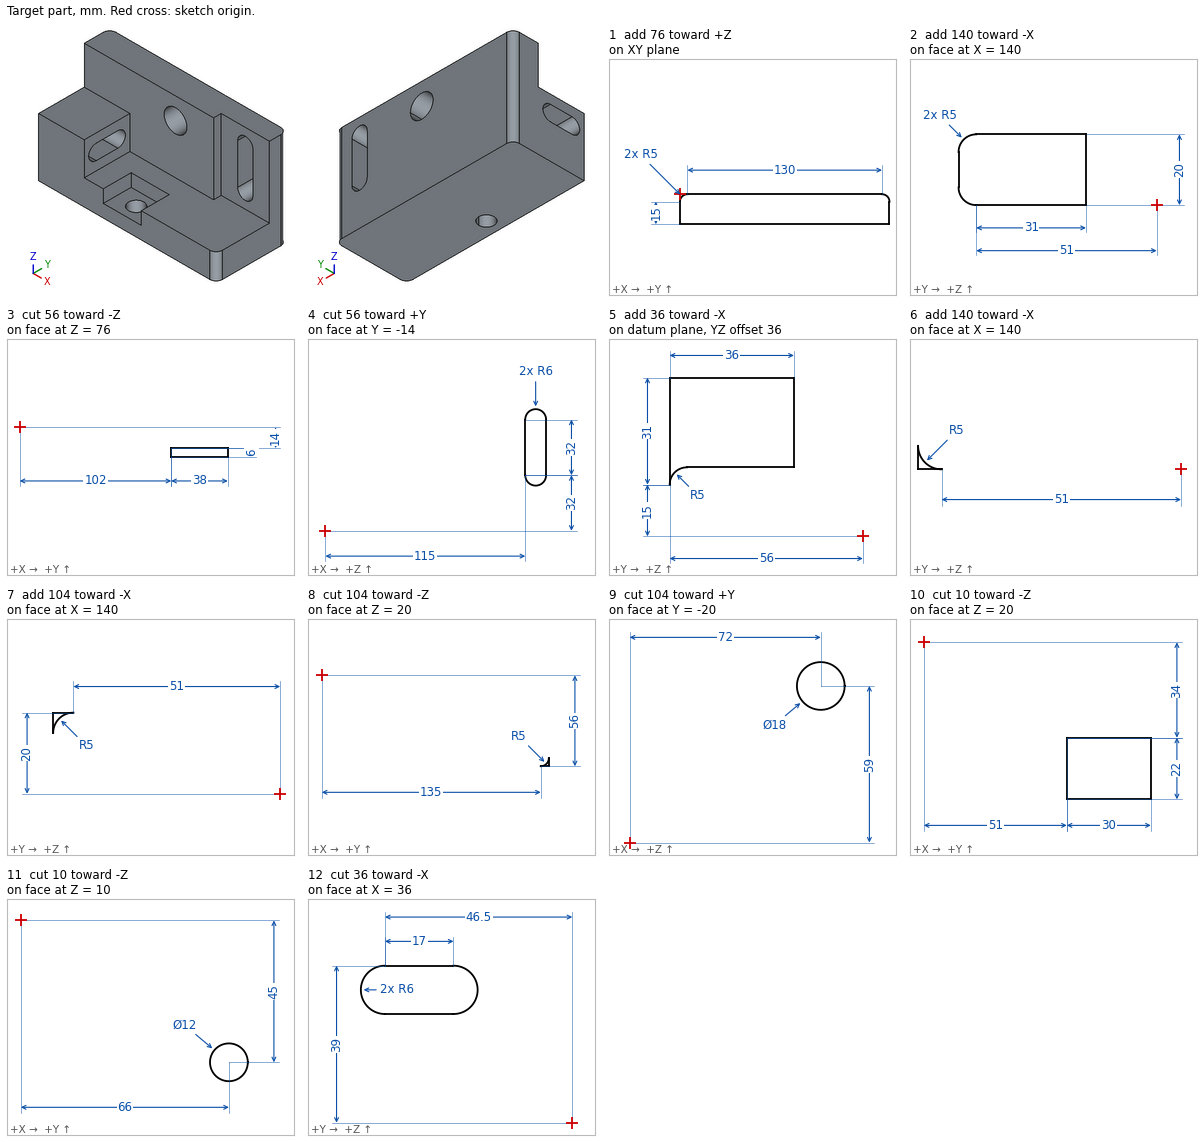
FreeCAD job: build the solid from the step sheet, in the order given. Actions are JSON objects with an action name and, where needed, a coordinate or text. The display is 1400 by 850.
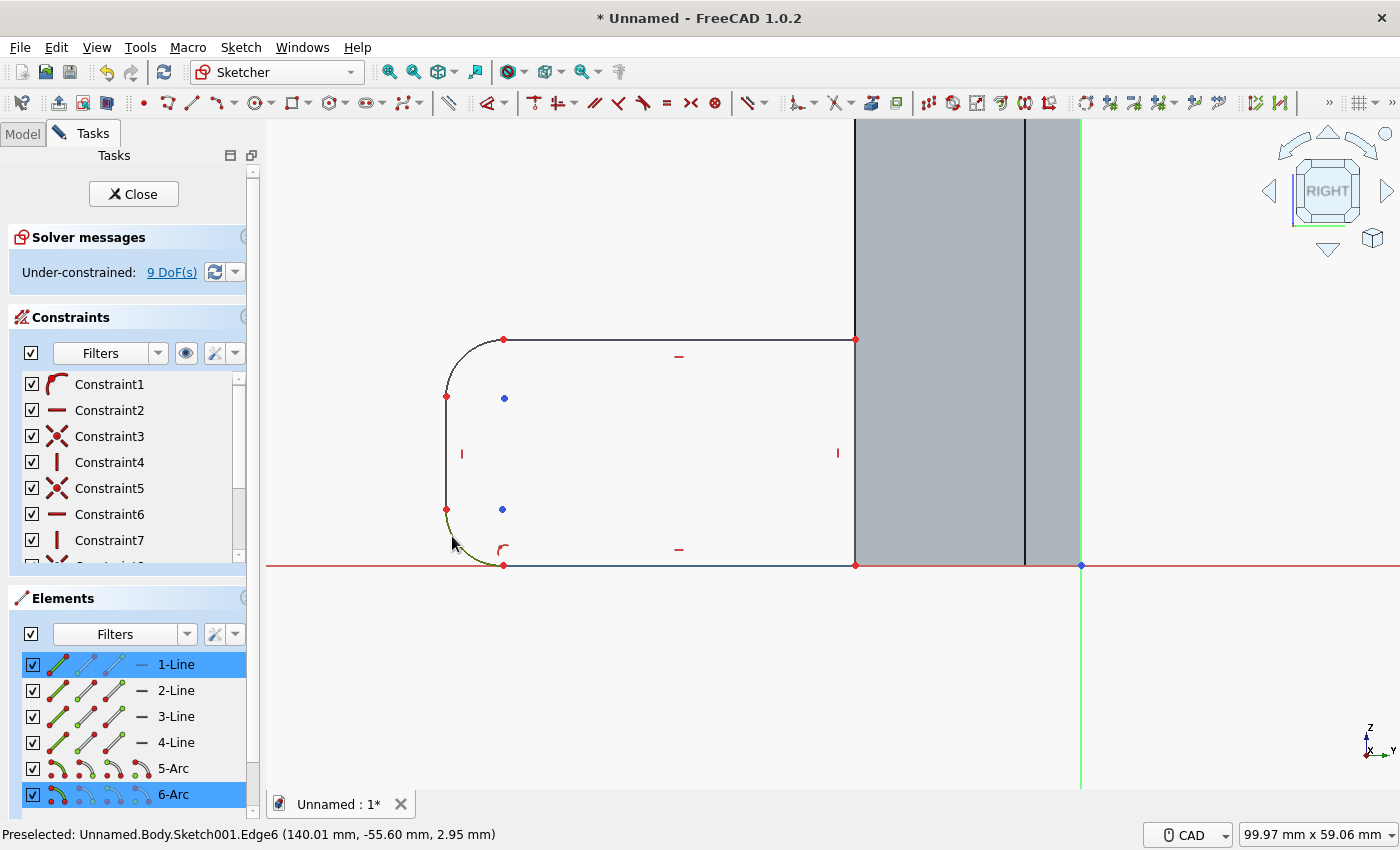
{"action": "key", "text": "t"}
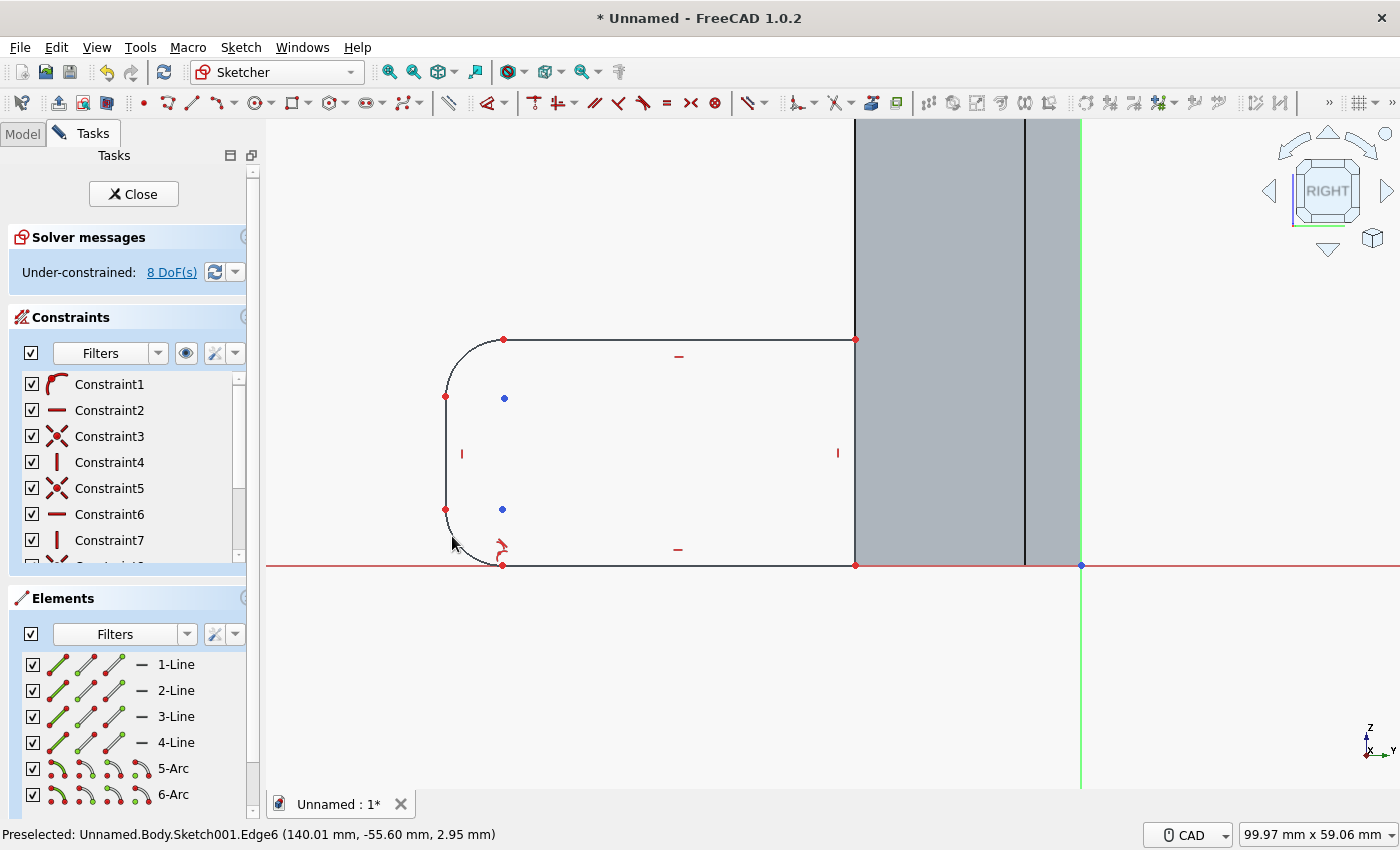
{"action": "left_click", "coordinate": [749, 340]}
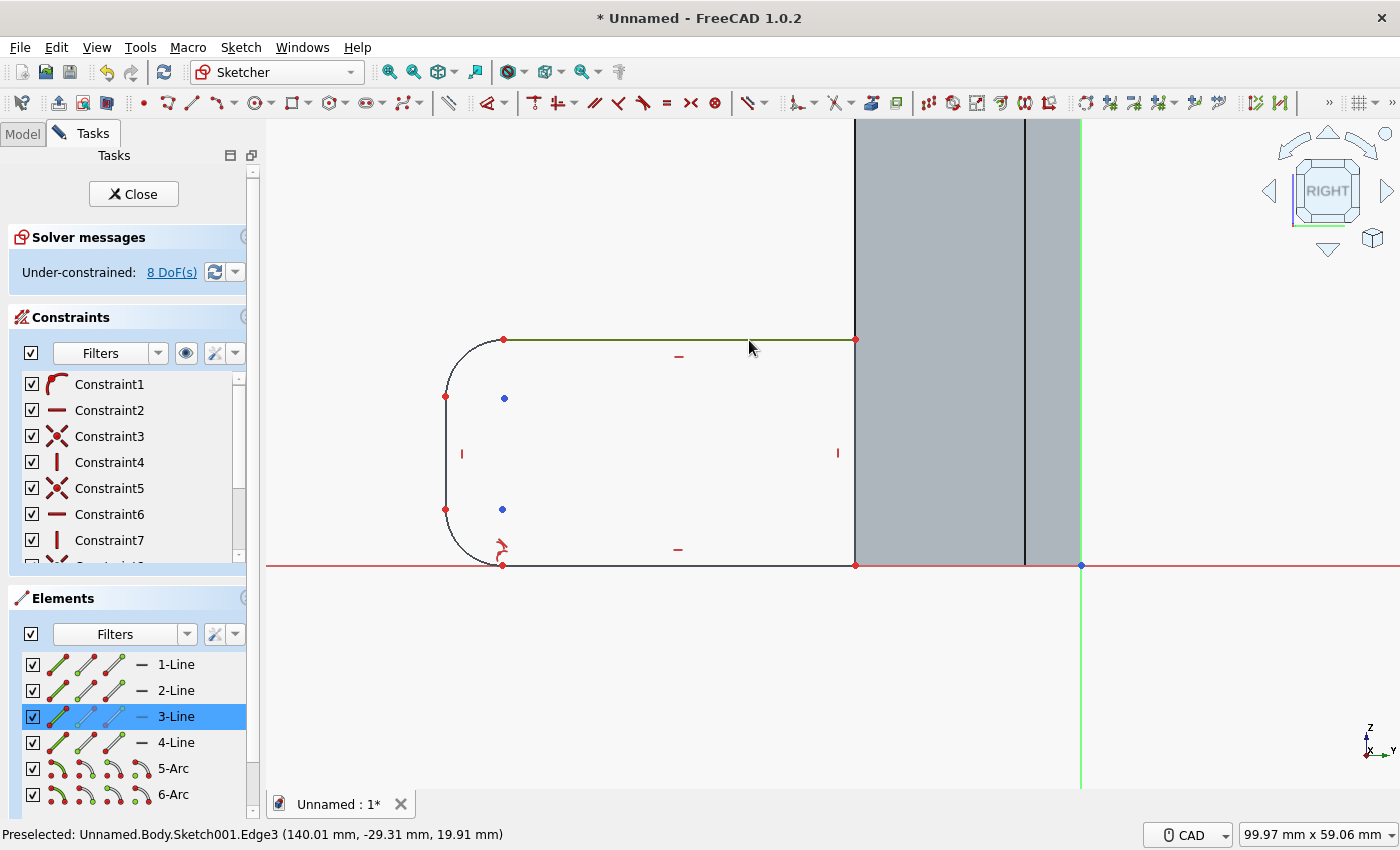
{"action": "left_click", "coordinate": [477, 347]}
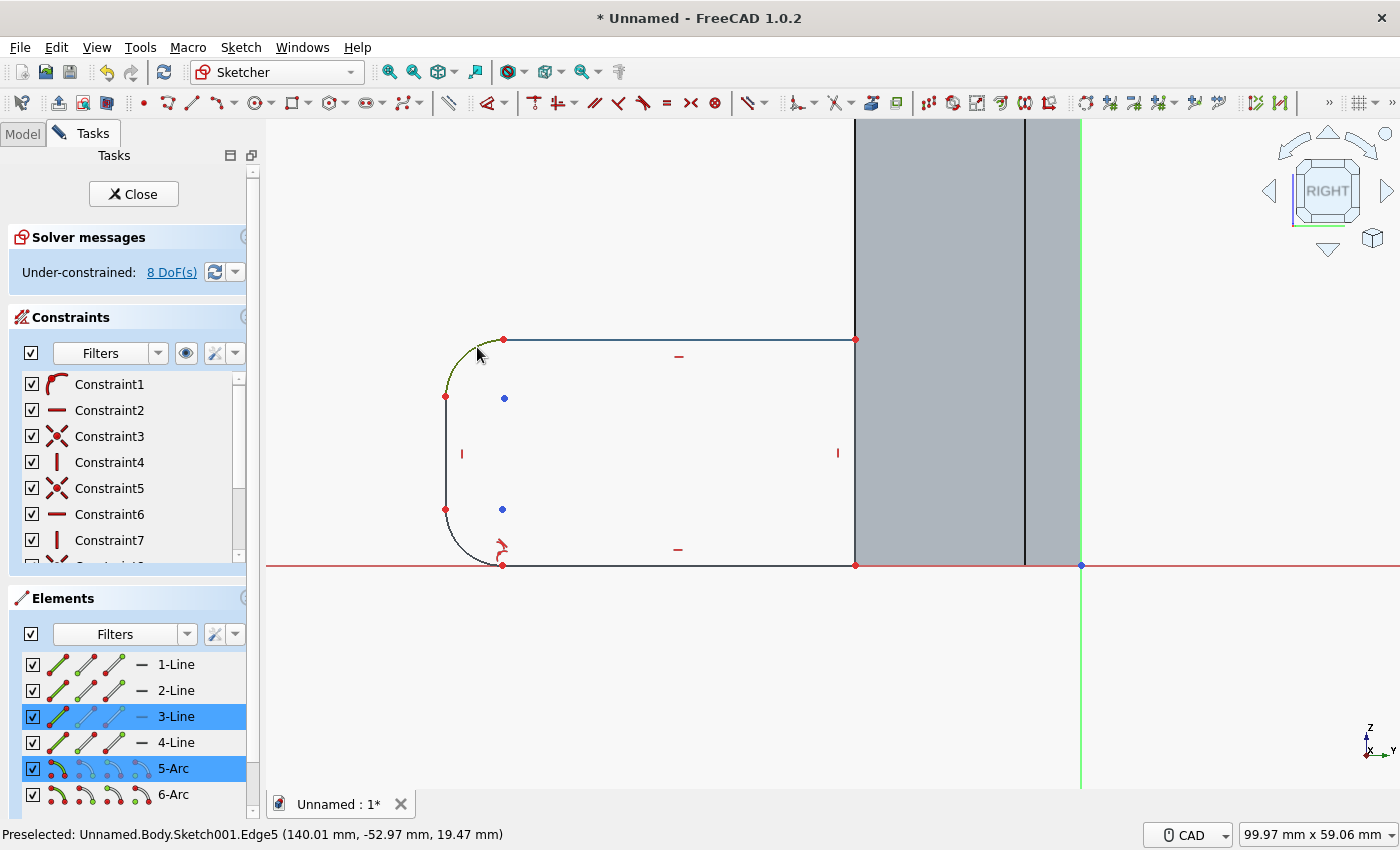
{"action": "left_click", "coordinate": [644, 104]}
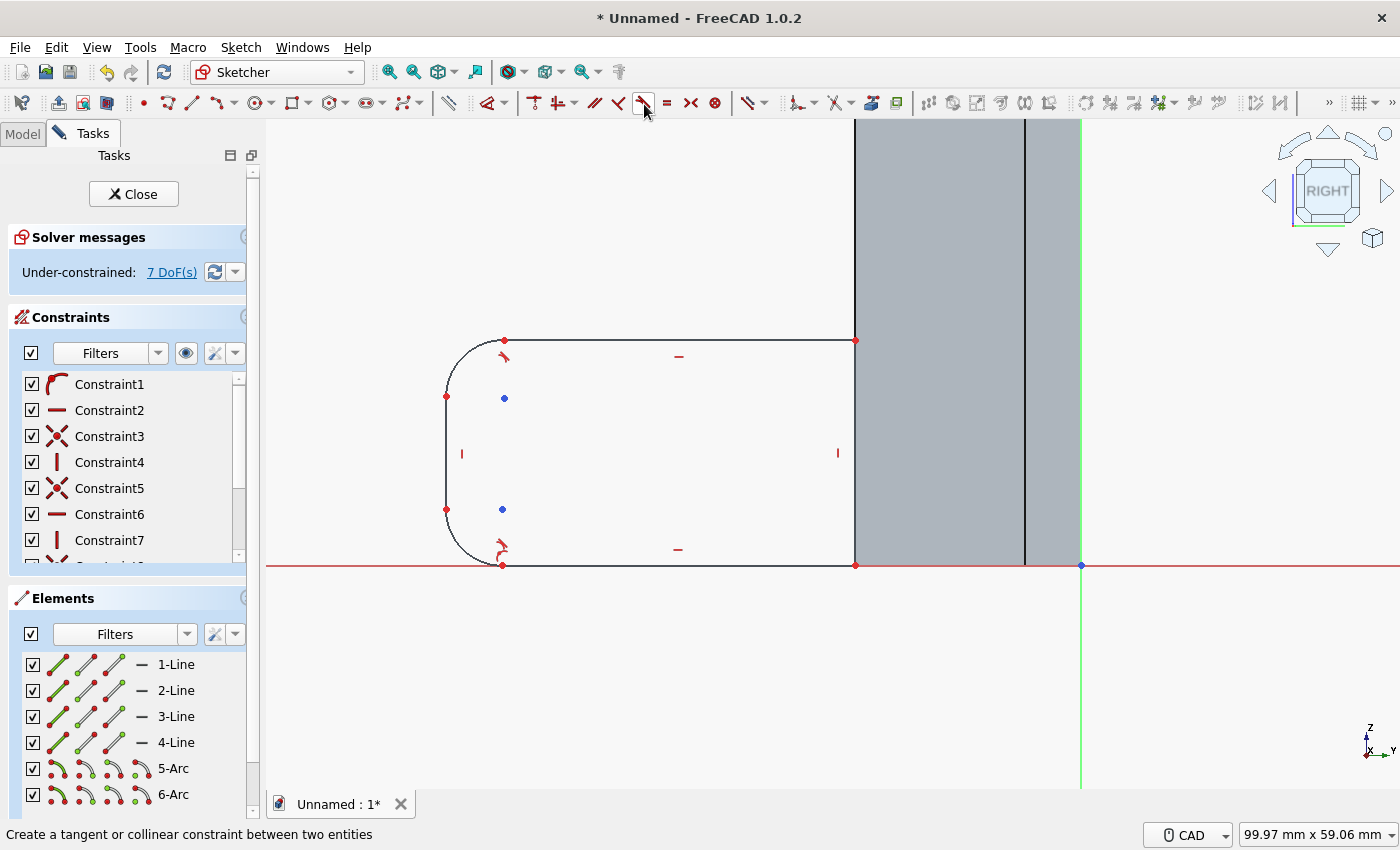
{"action": "left_click", "coordinate": [446, 431]}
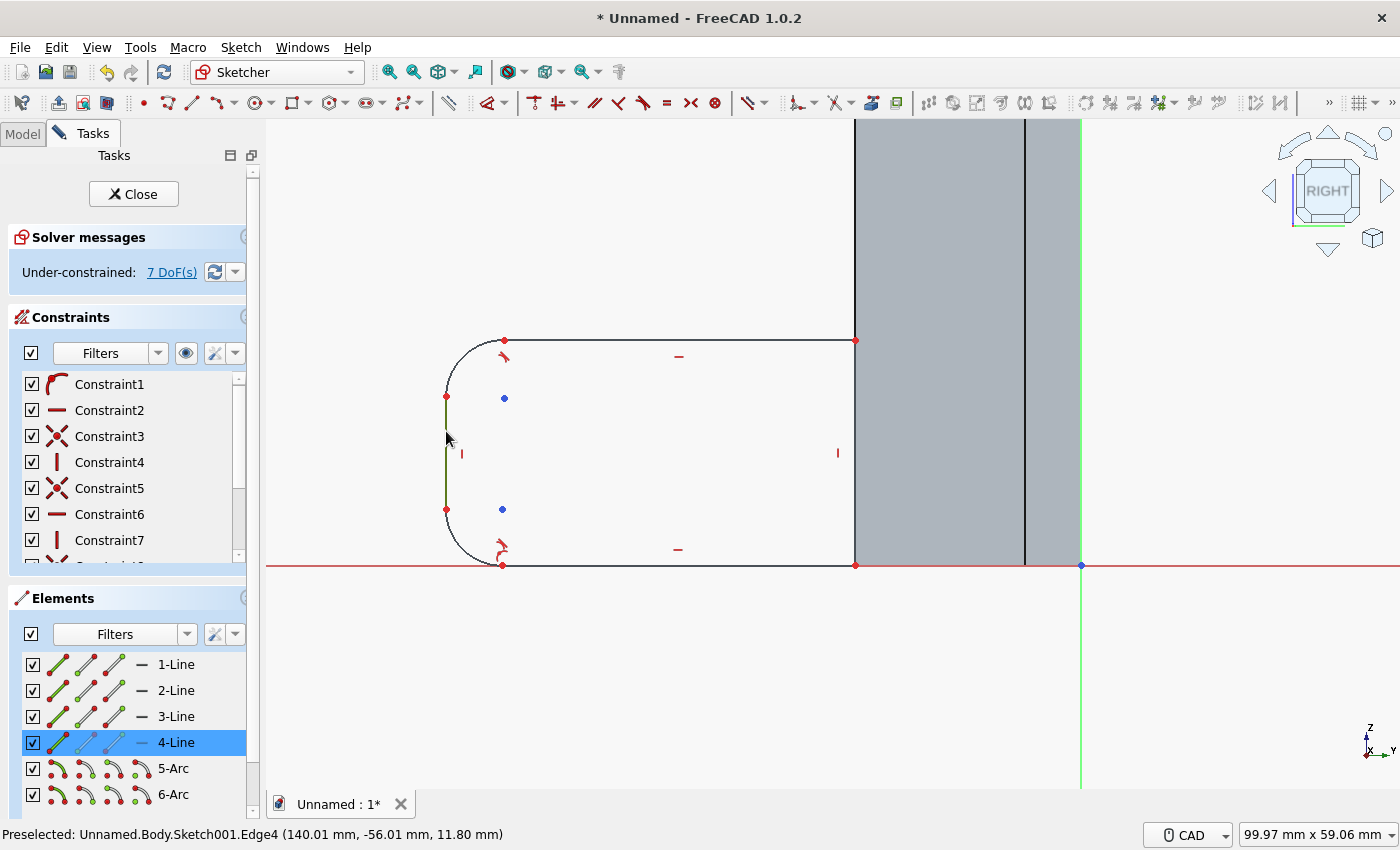
{"action": "left_click", "coordinate": [478, 346]}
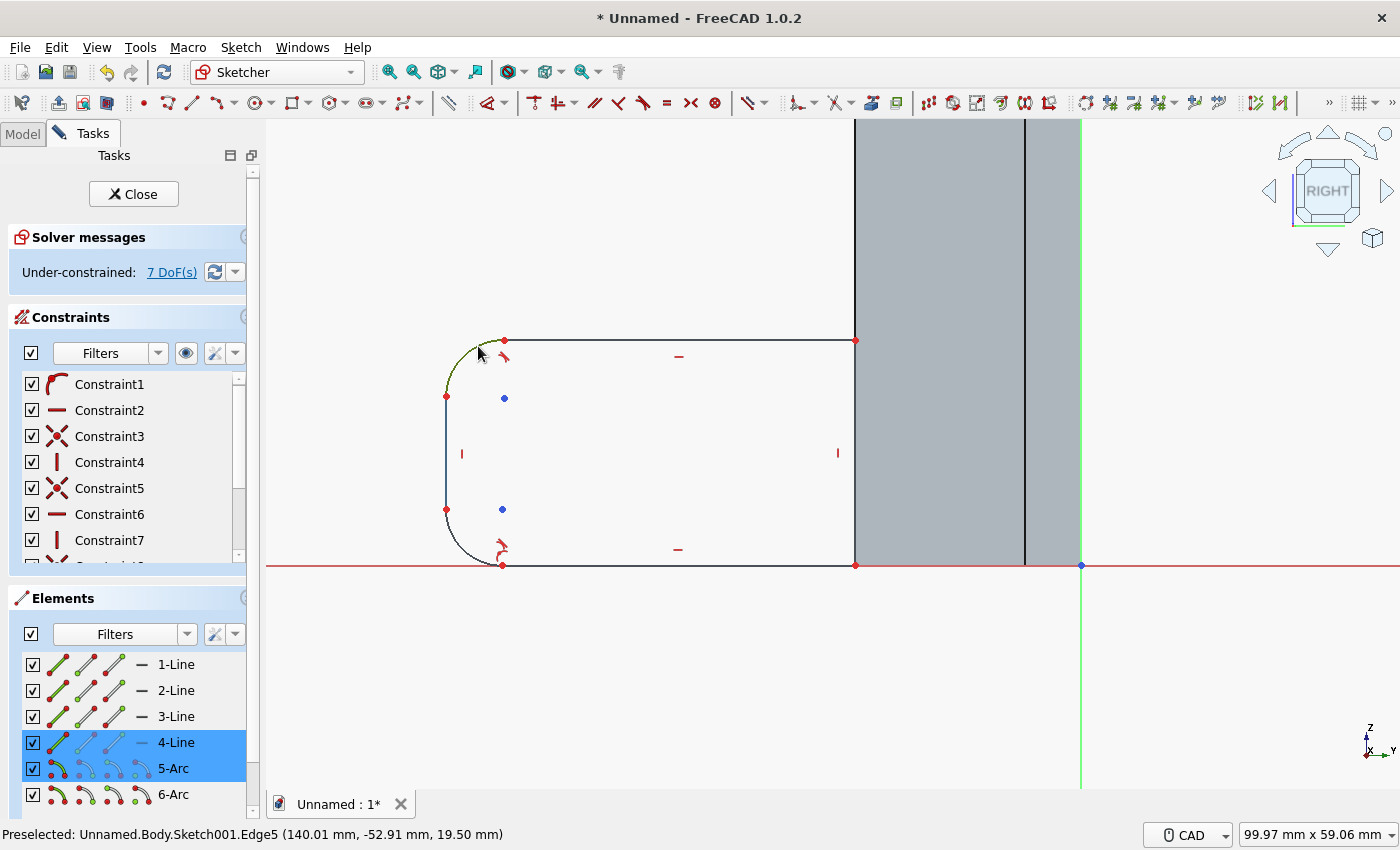
{"action": "left_click", "coordinate": [644, 104]}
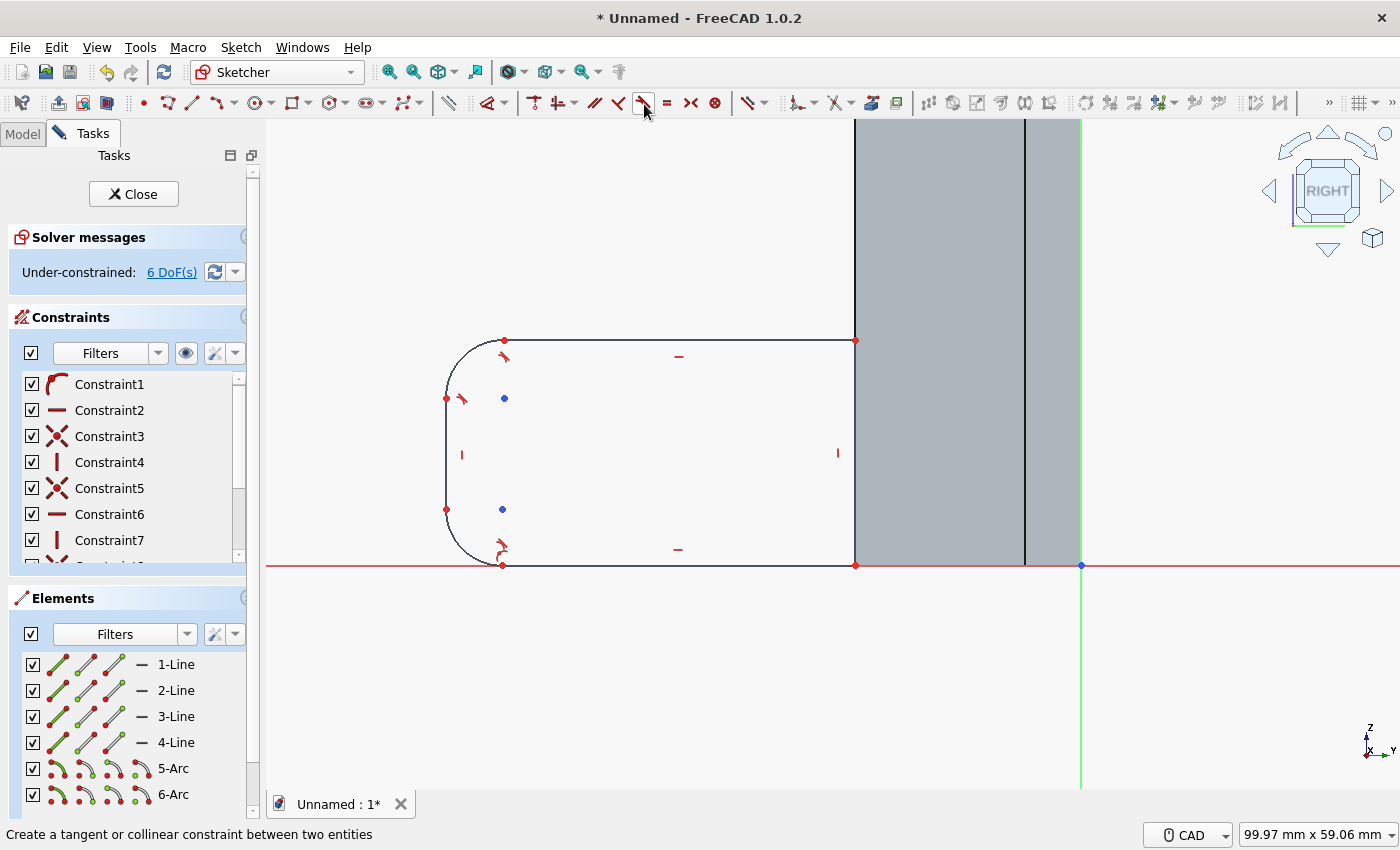
{"action": "left_click", "coordinate": [446, 432]}